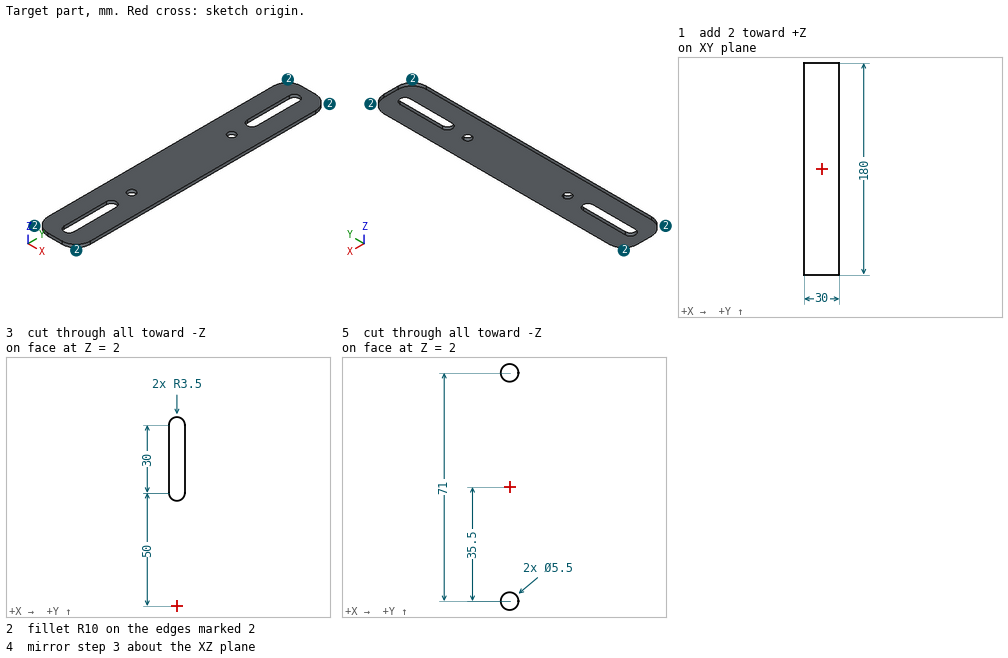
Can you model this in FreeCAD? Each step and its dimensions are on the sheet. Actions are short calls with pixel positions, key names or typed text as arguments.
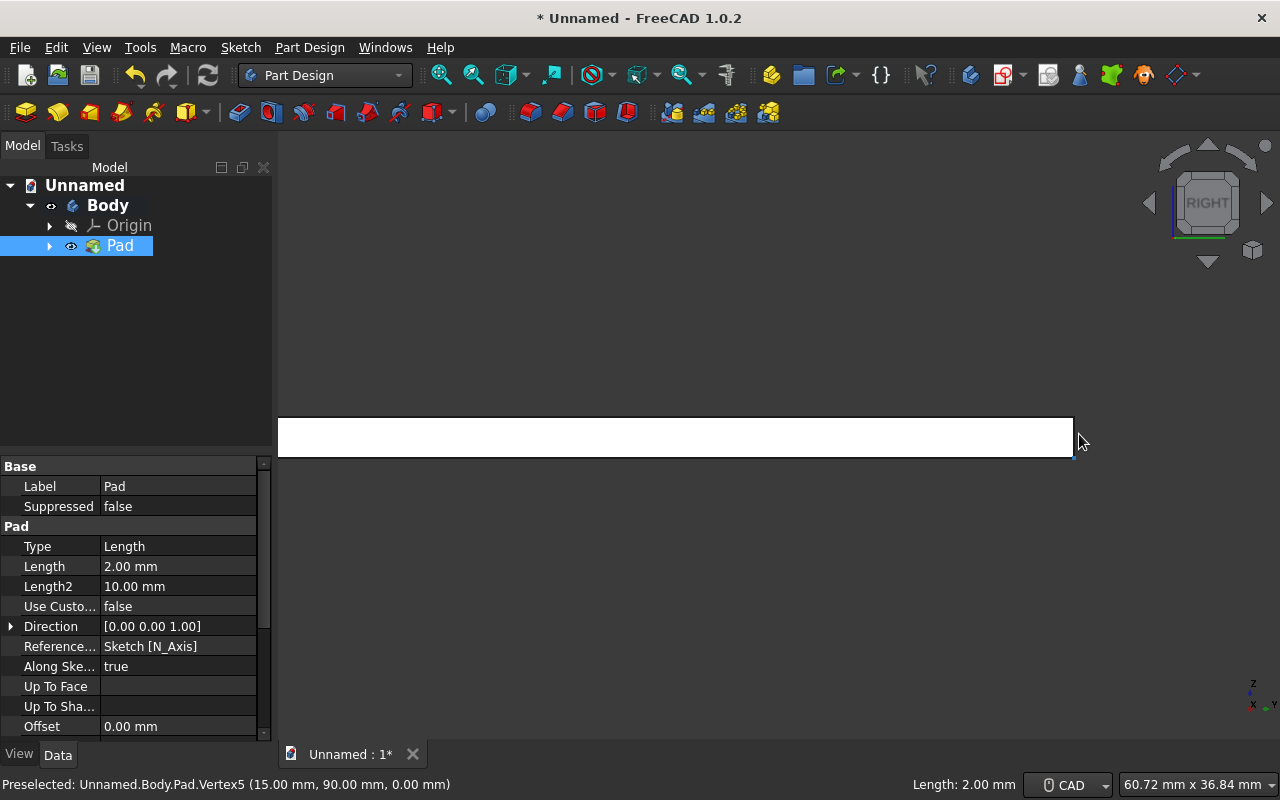
click(1074, 437, ctrl)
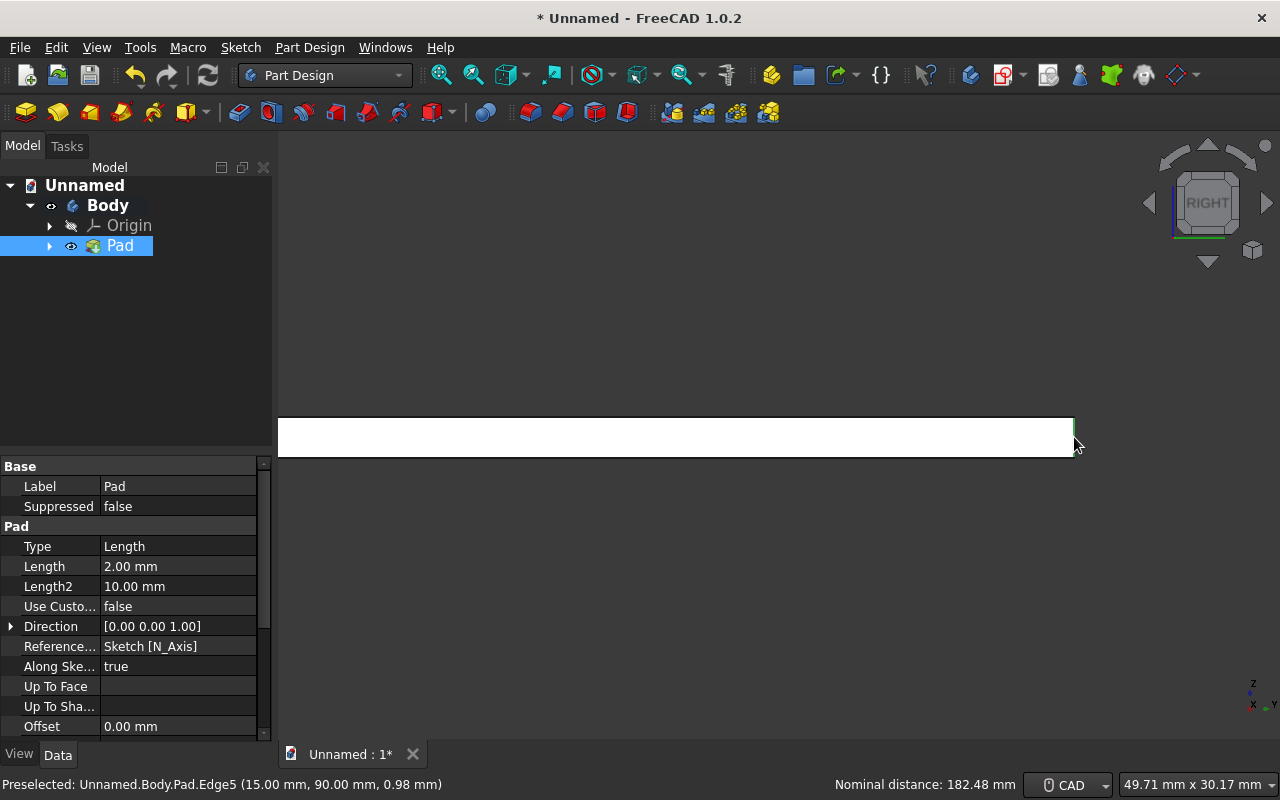
key(v)
key(f)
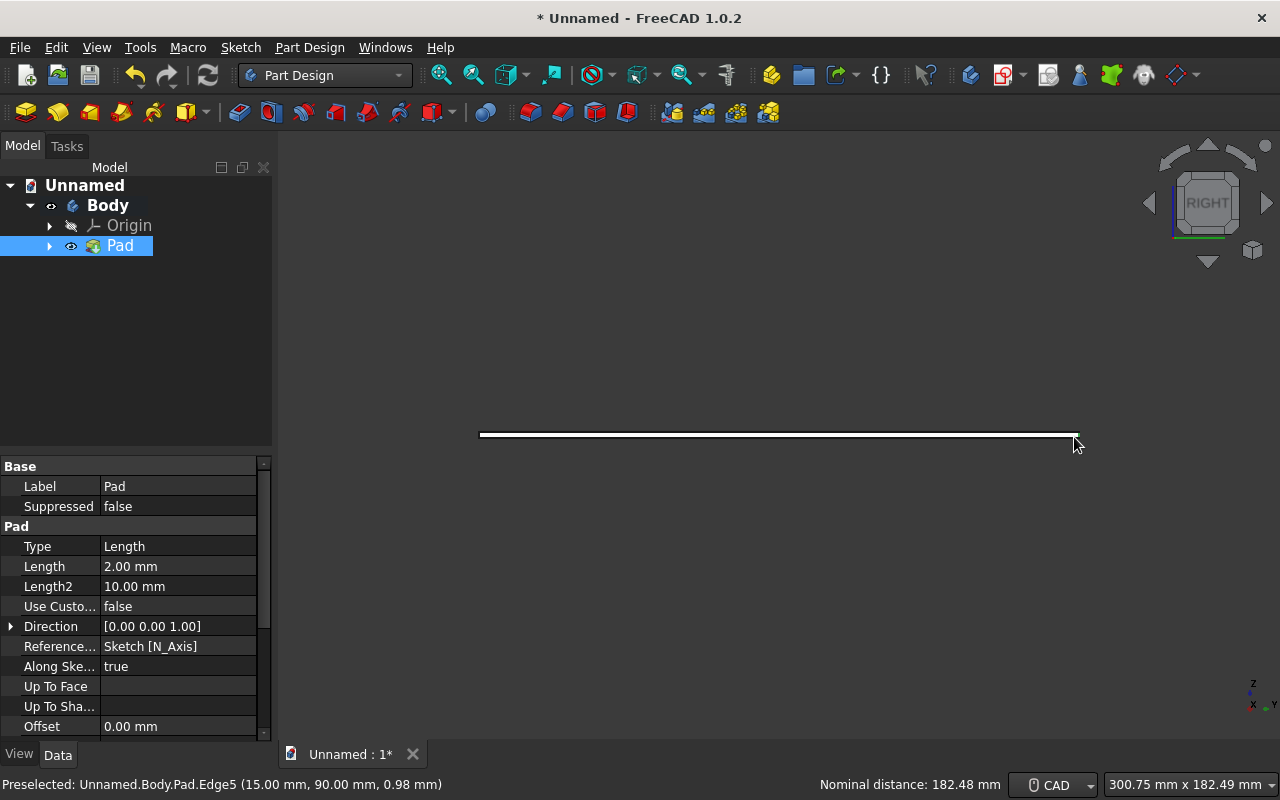
key(5)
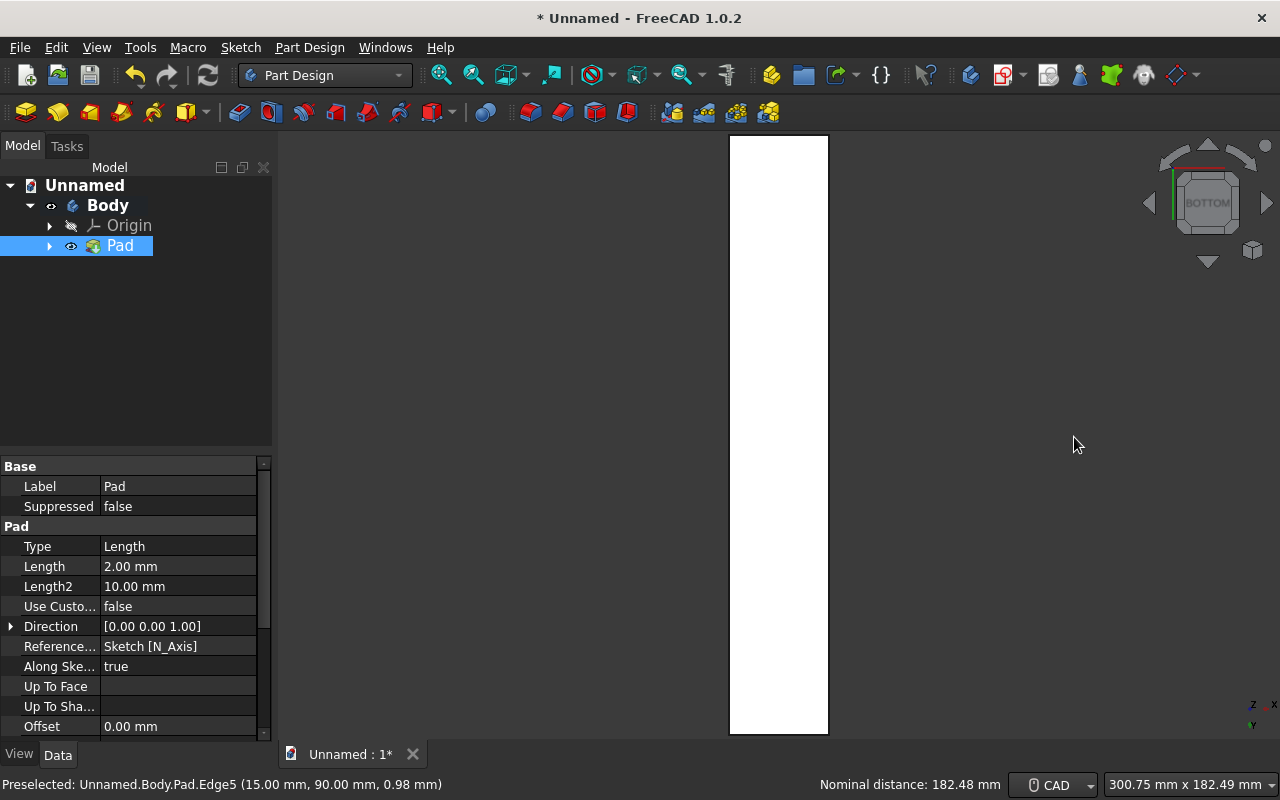
key(4)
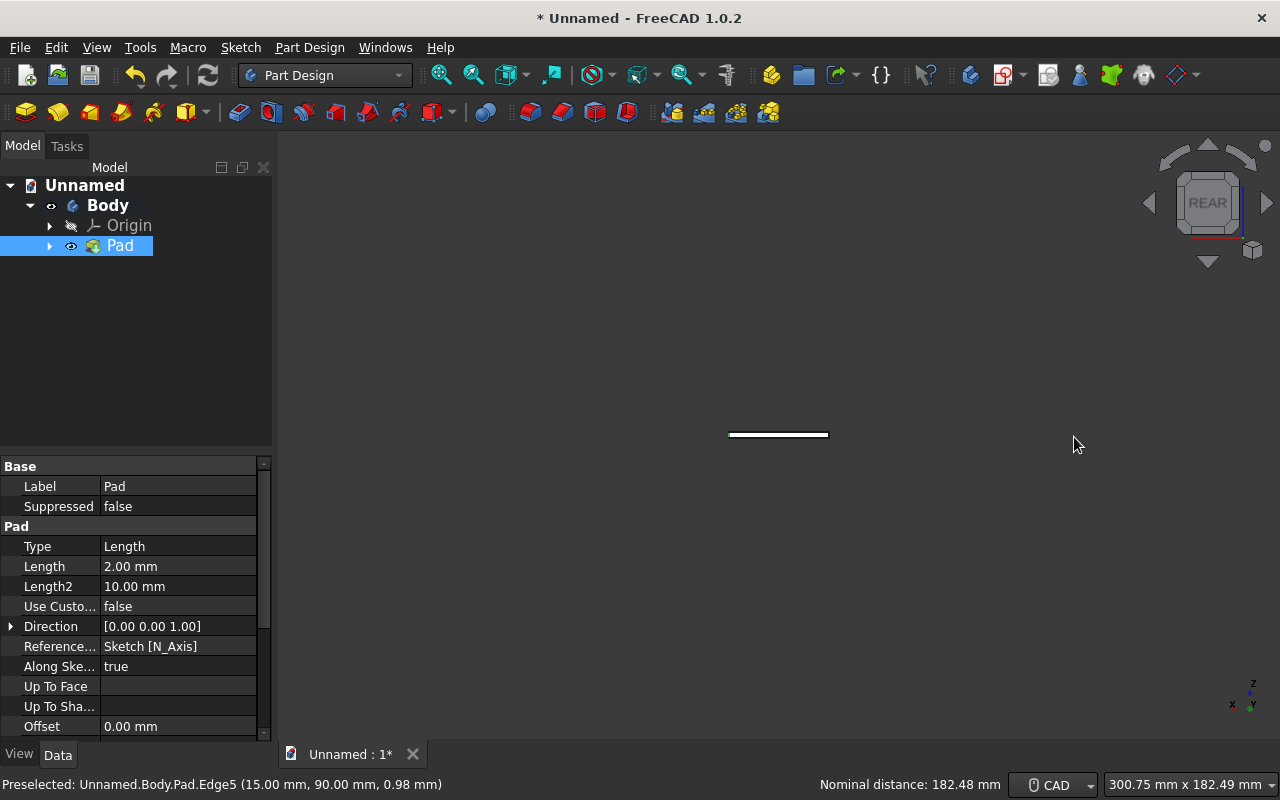
click(442, 76)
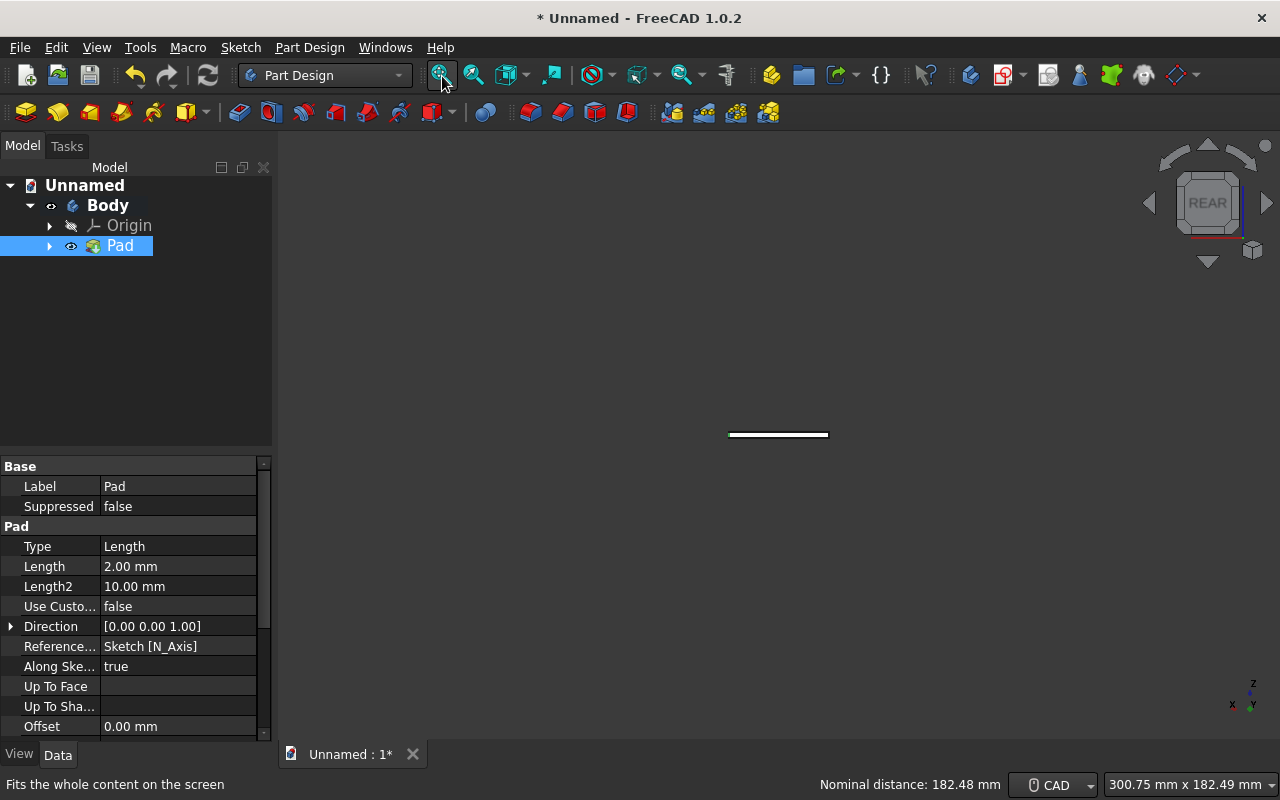
scroll(829, 434, up, 9)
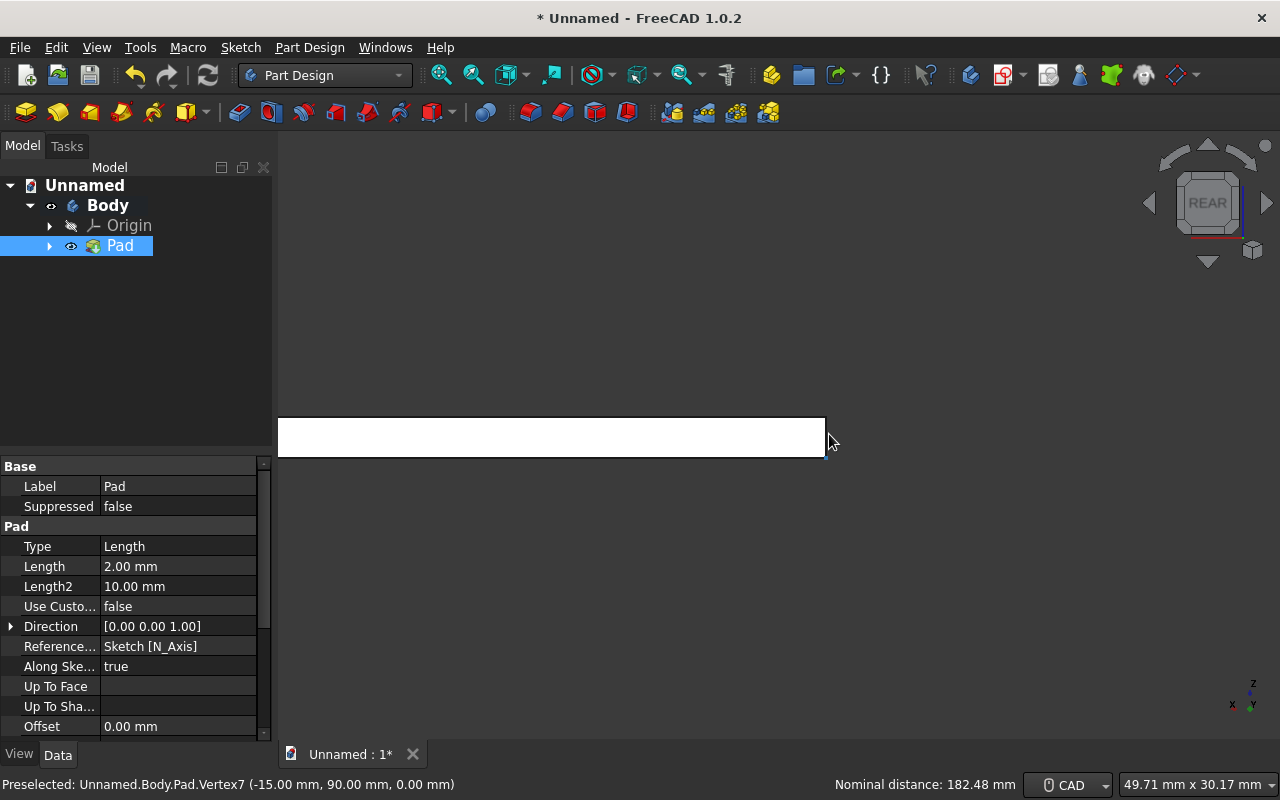
click(826, 437, ctrl)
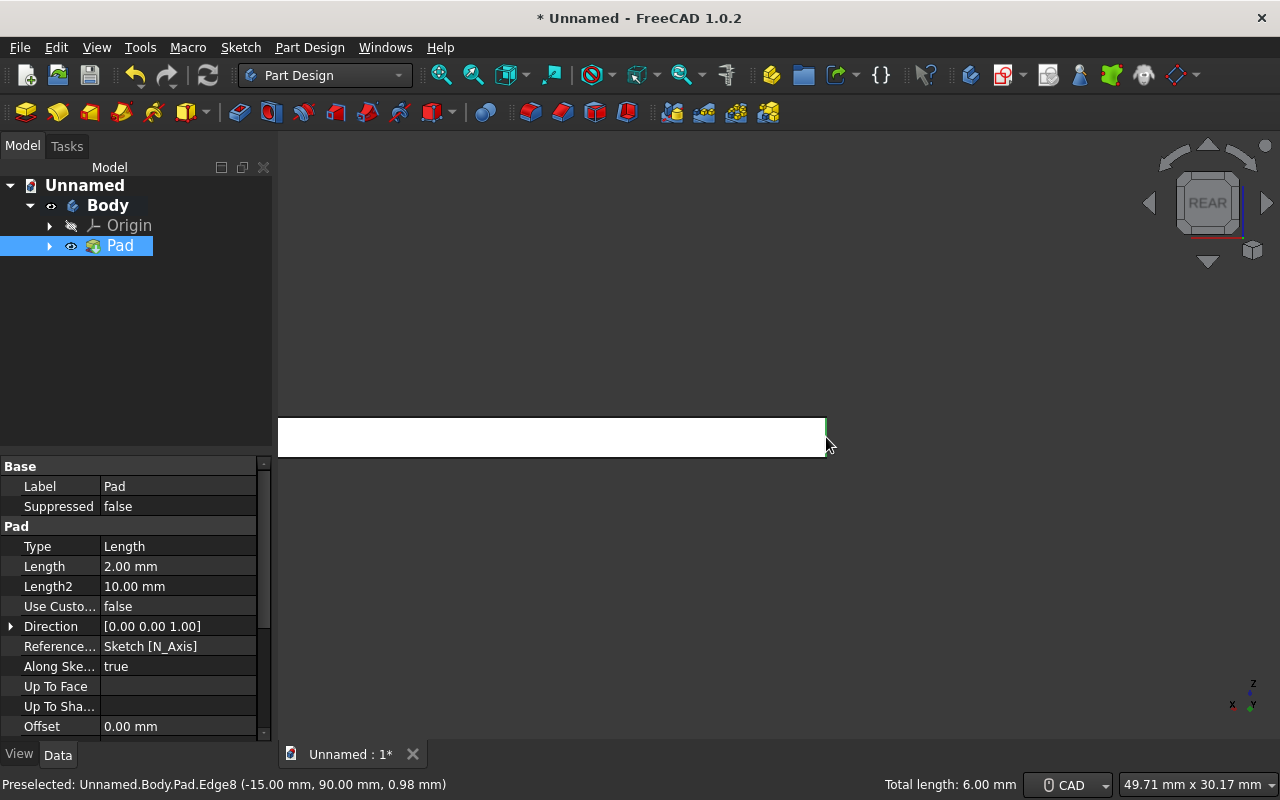
key(v)
key(f)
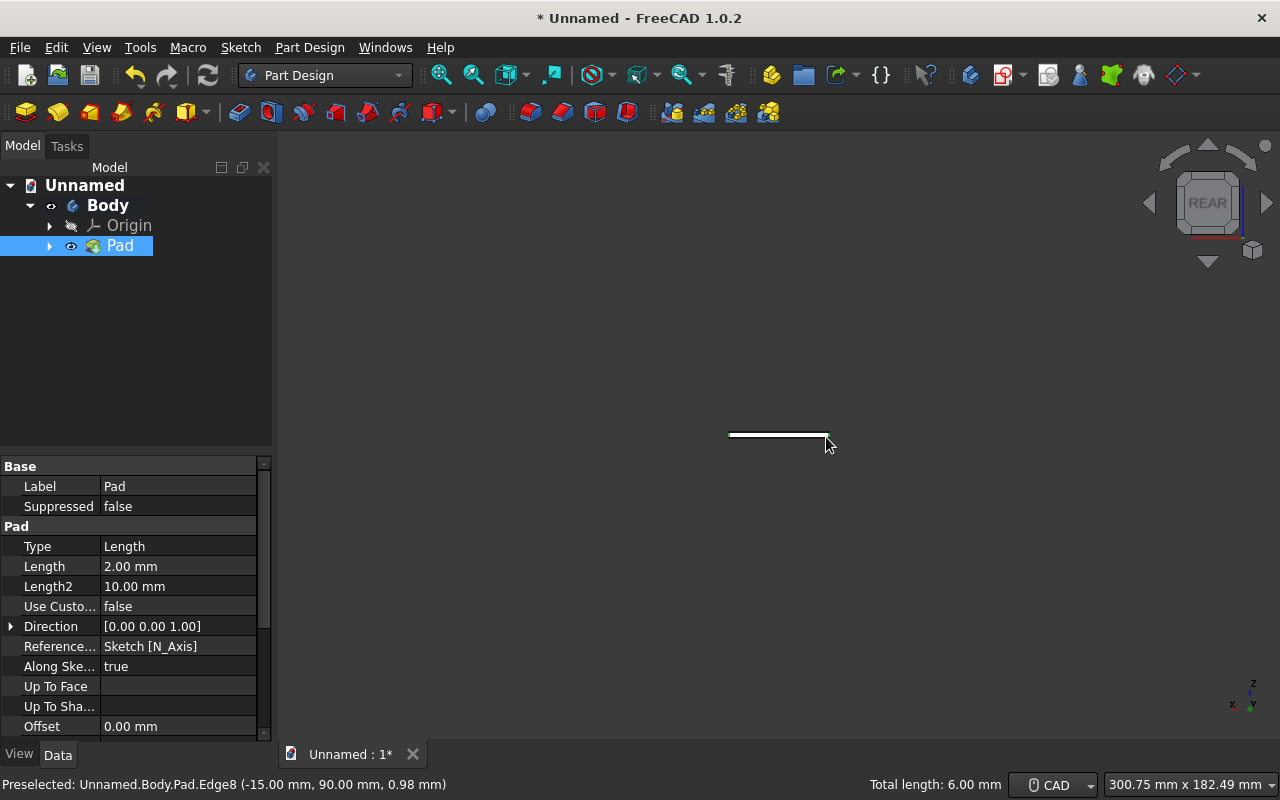
key(6)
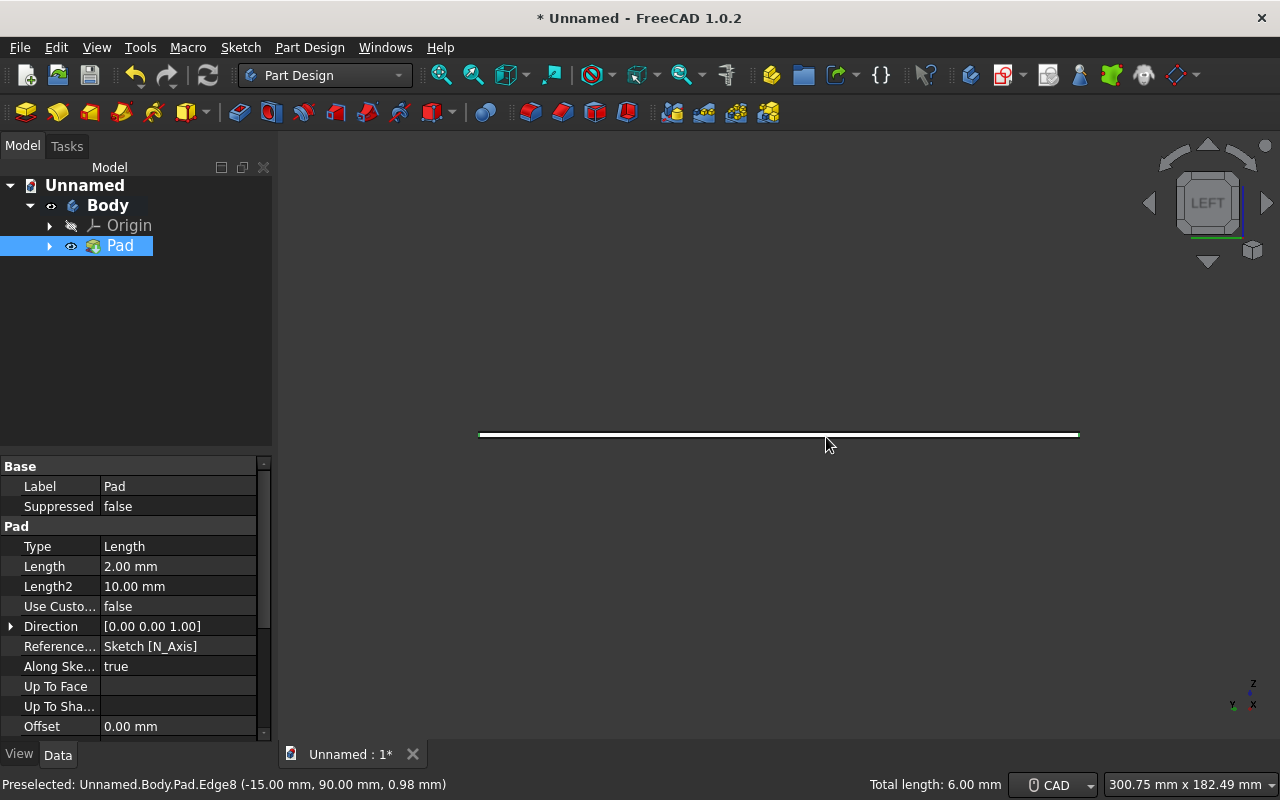
scroll(1079, 434, up, 9)